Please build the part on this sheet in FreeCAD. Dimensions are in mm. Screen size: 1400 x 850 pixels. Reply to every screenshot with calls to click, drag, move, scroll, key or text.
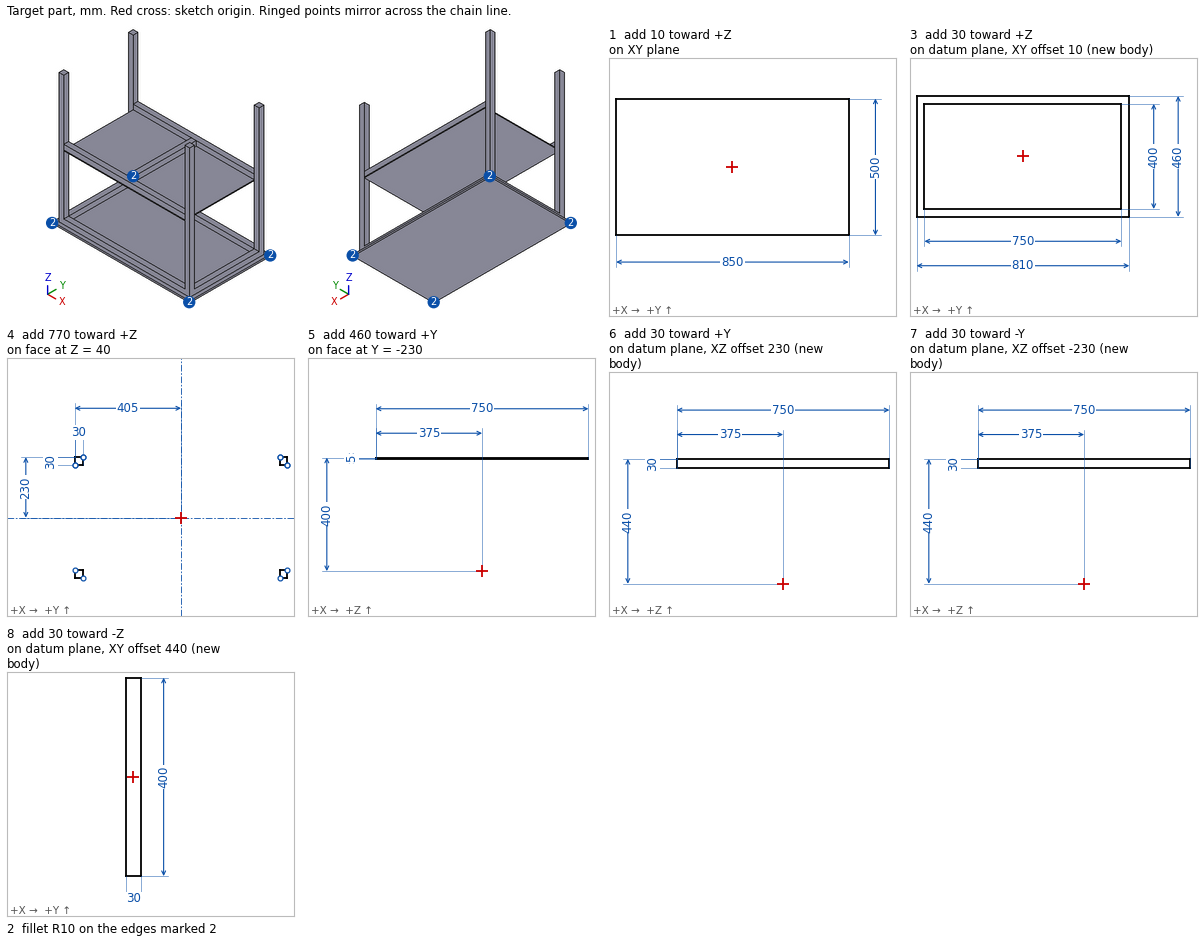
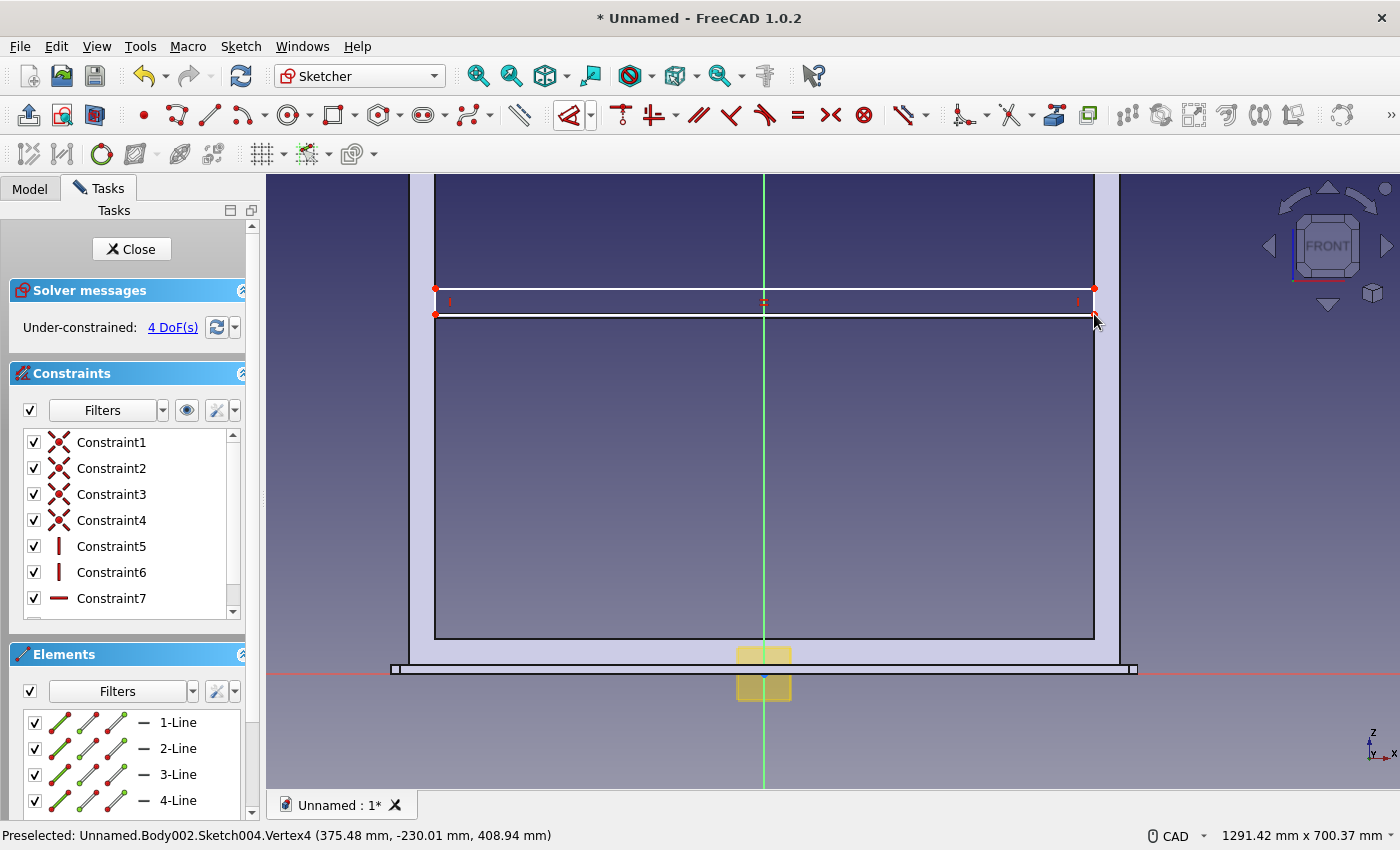
scroll(435, 299, up, 3)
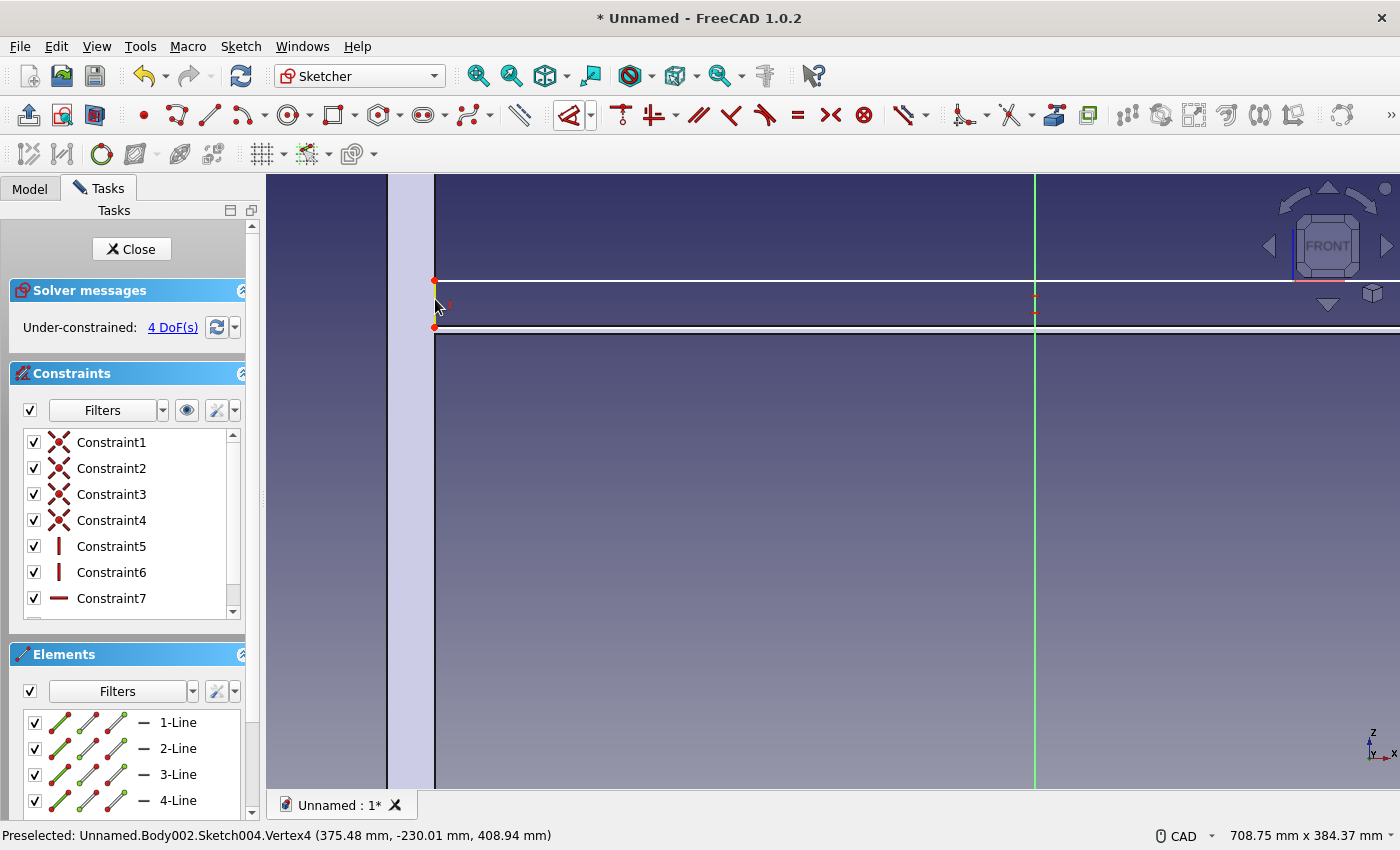
click(435, 300)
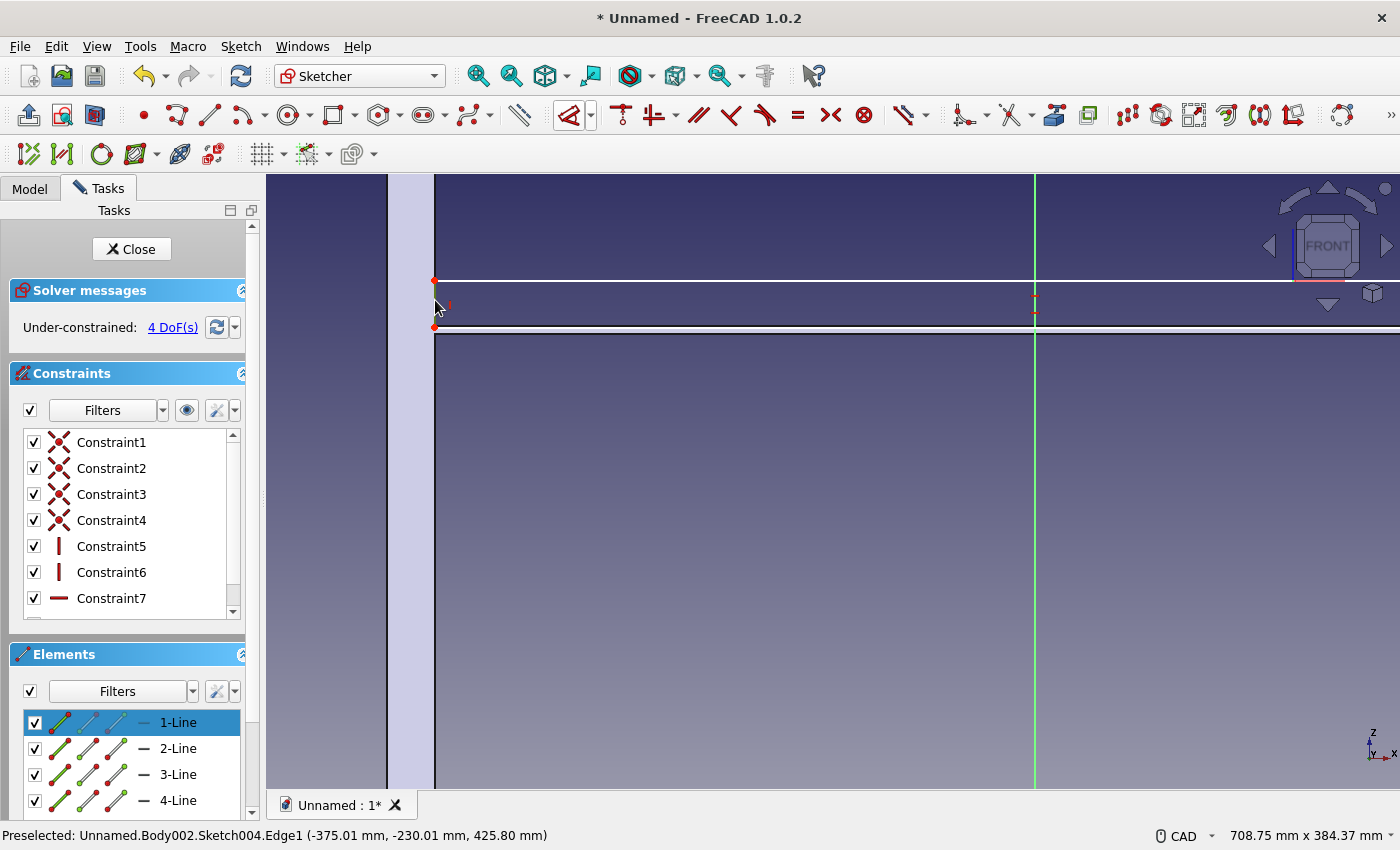
click(590, 116)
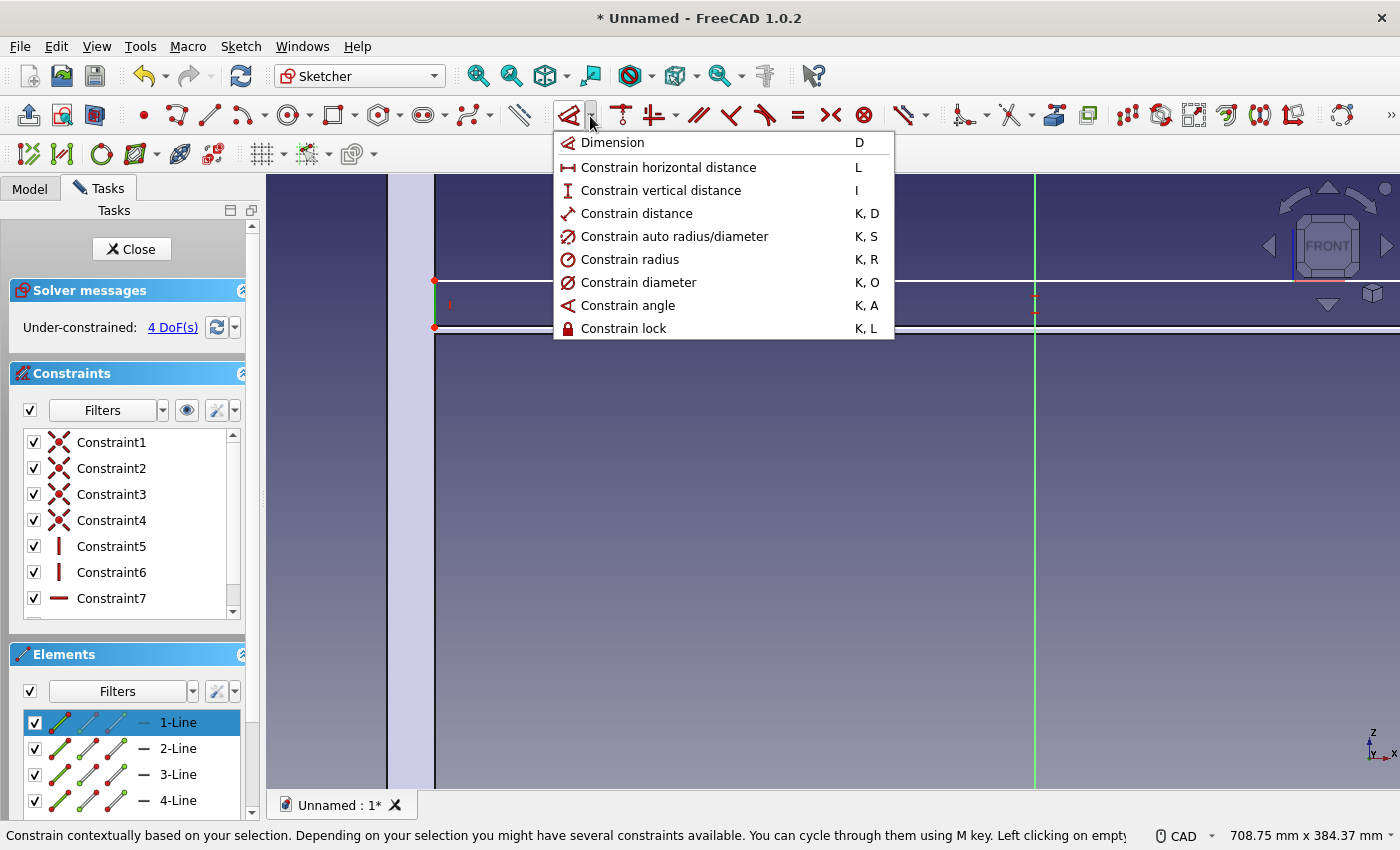
click(724, 190)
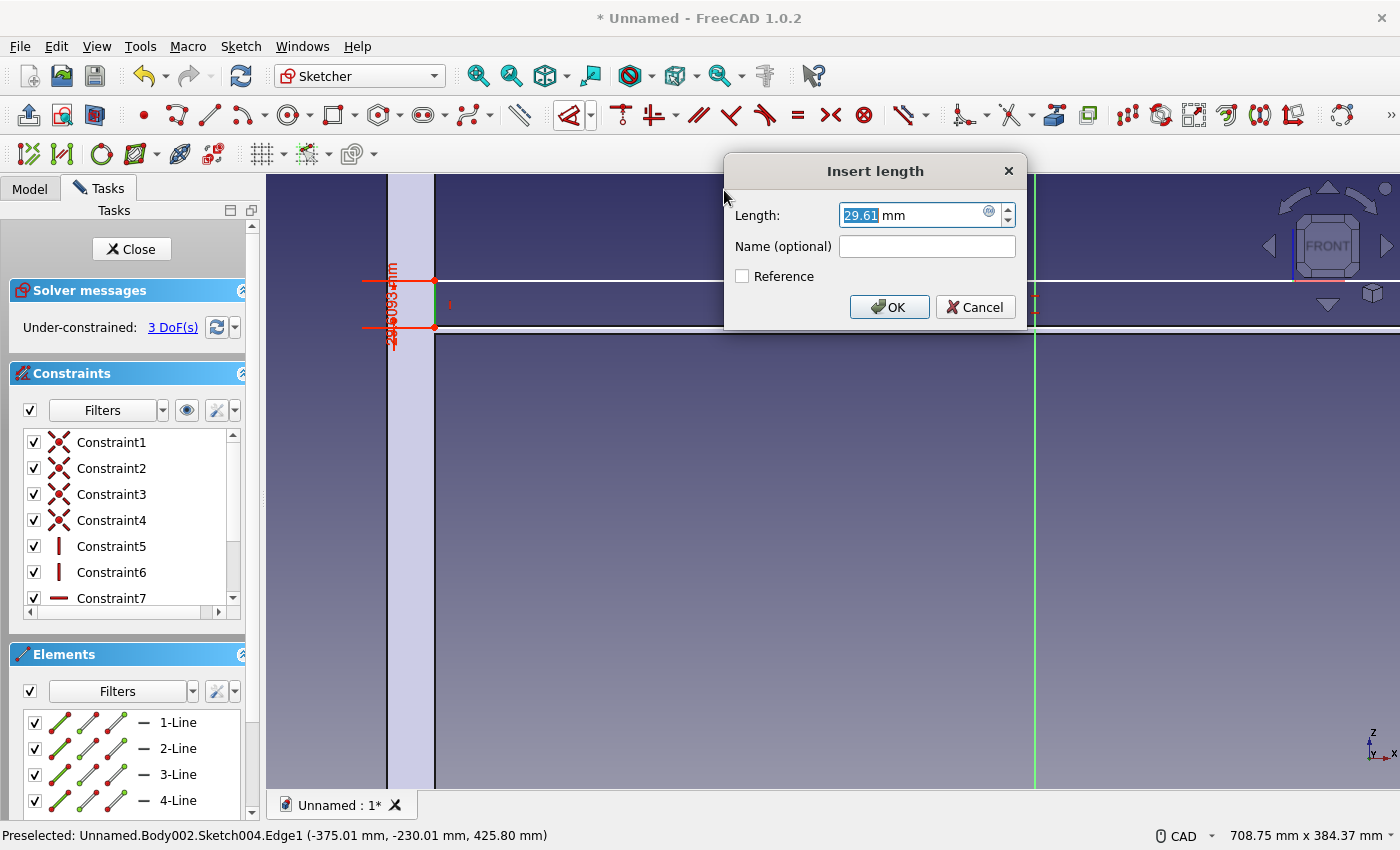
text(30)
key(Return)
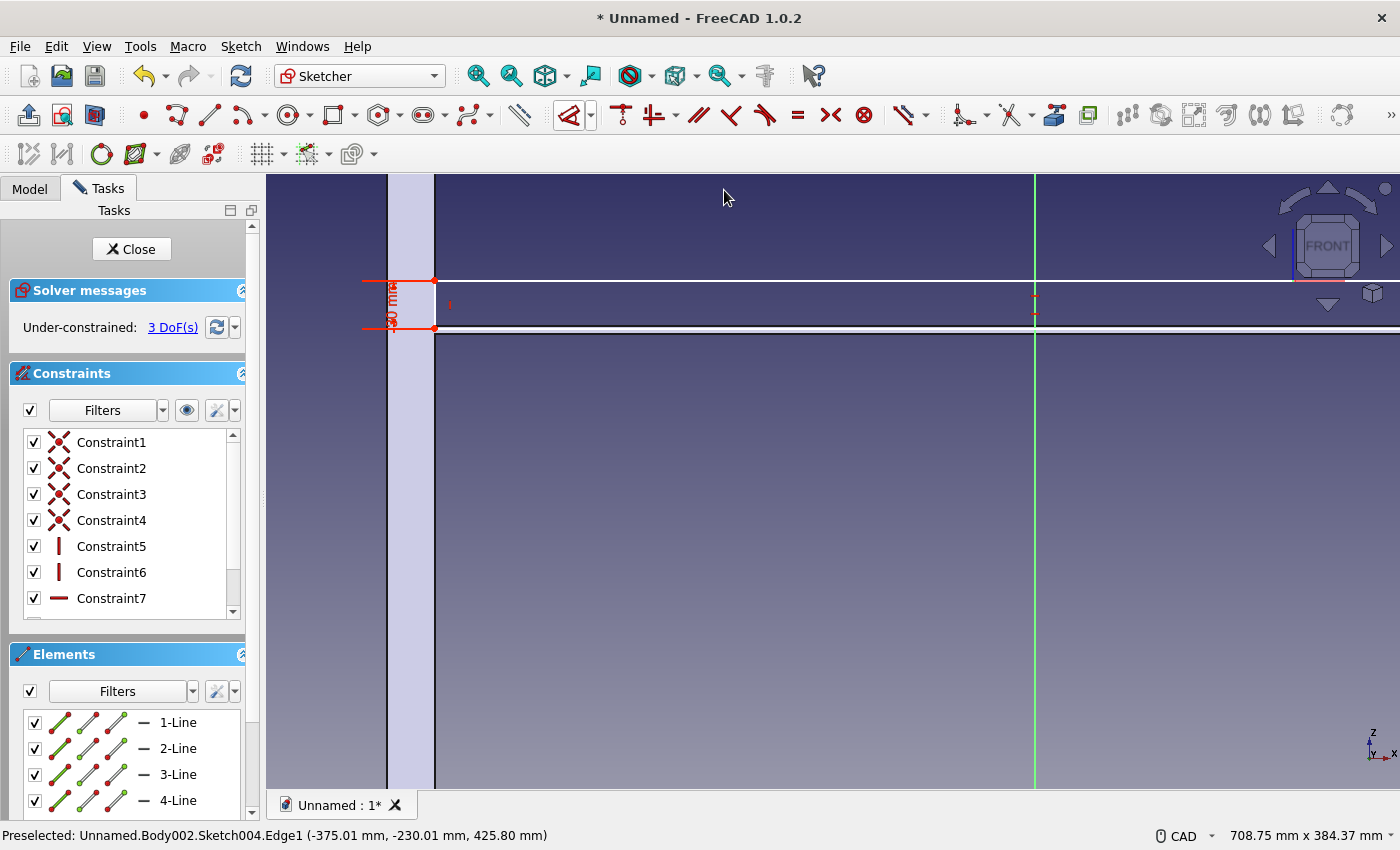
click(795, 328)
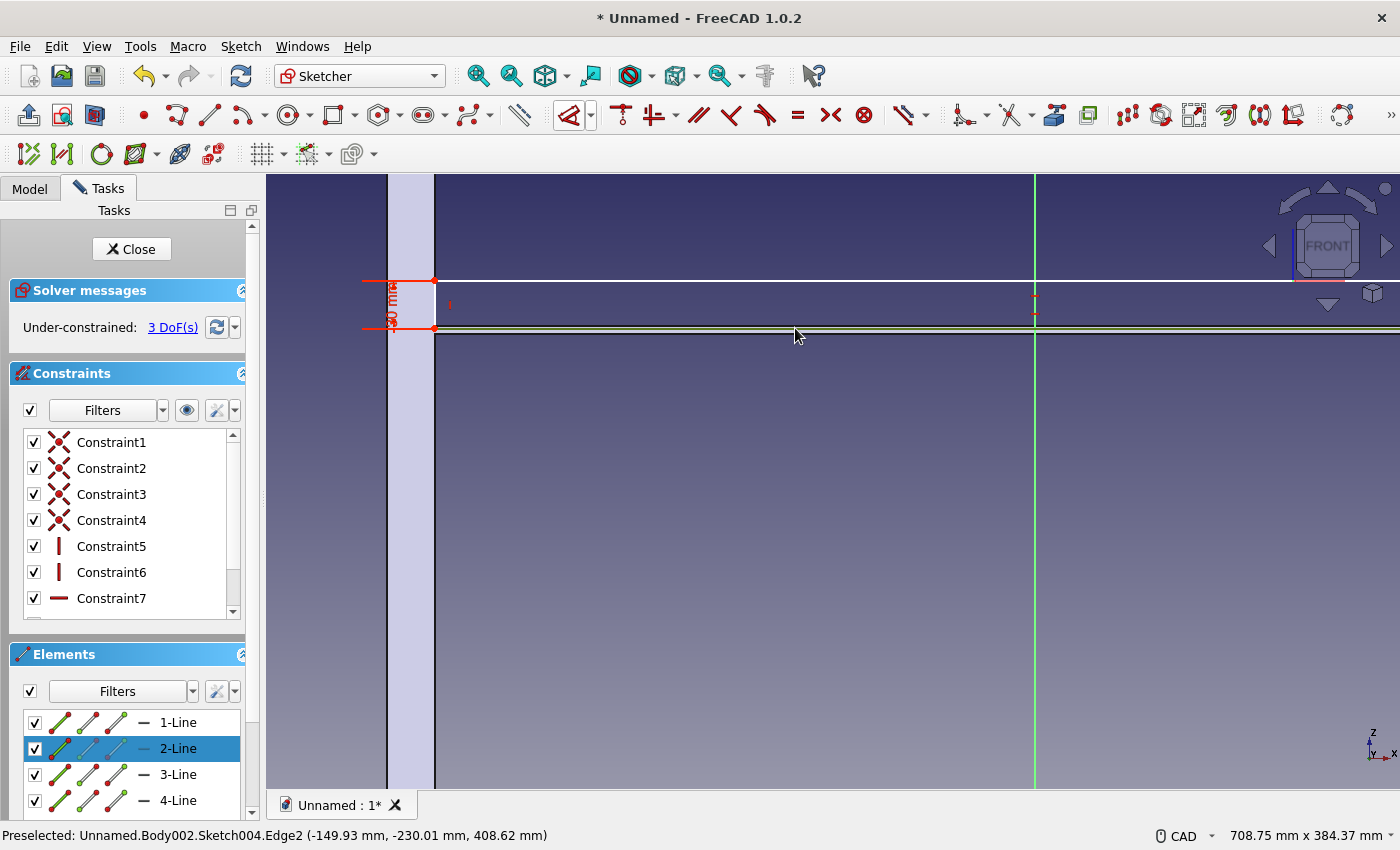
click(590, 116)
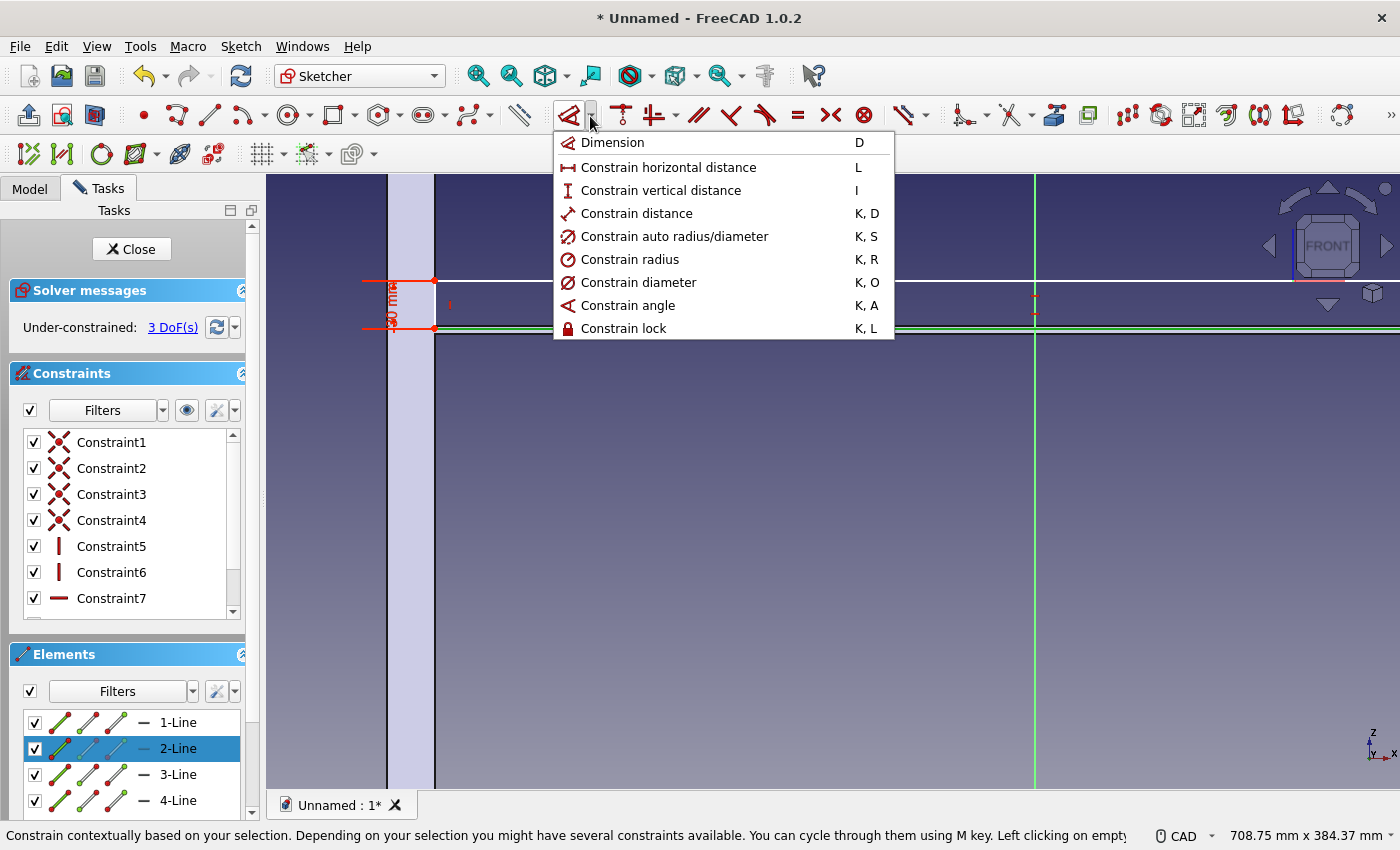
click(724, 168)